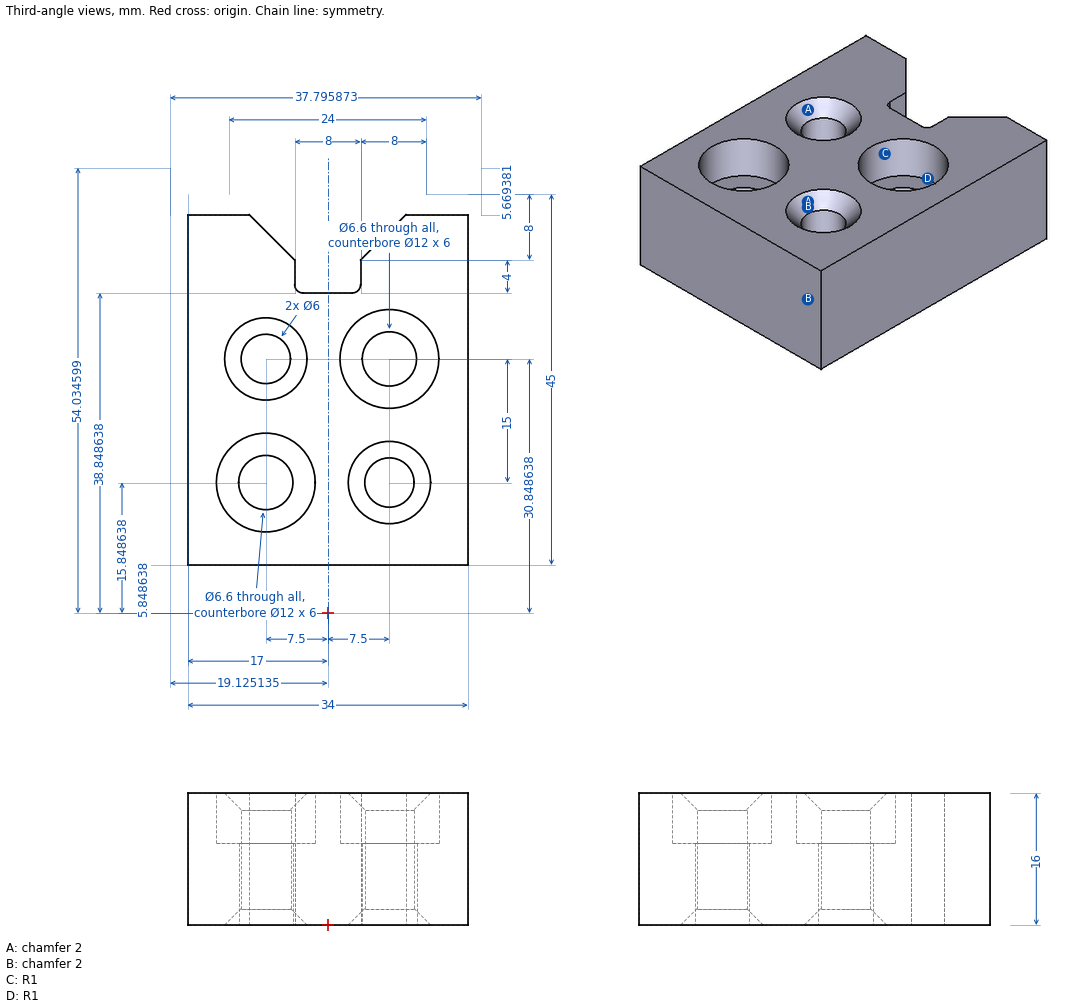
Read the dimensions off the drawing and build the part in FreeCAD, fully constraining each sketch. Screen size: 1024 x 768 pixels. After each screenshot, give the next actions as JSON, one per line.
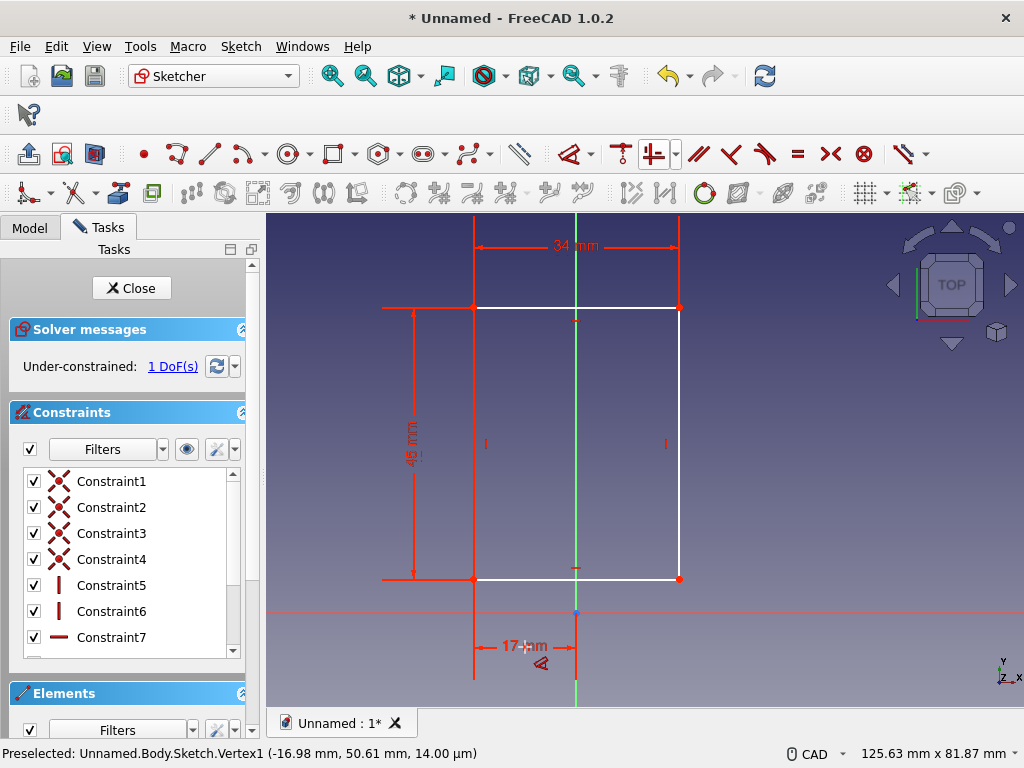
{"action": "left_click", "coordinate": [474, 580]}
{"action": "left_click", "coordinate": [440, 596]}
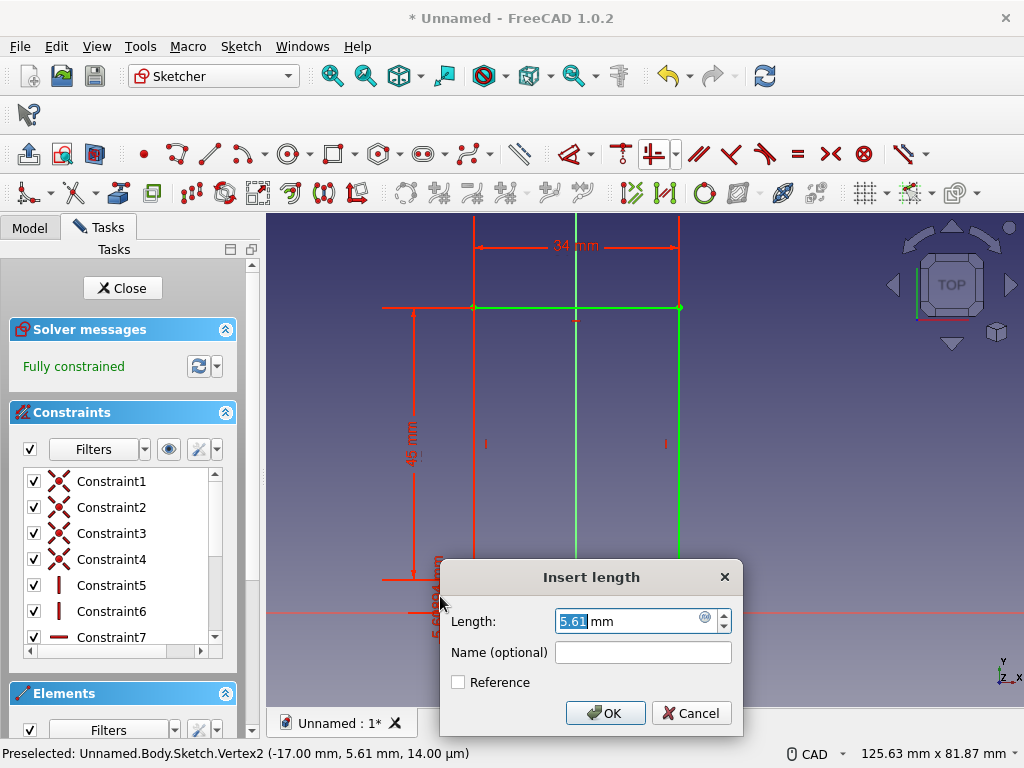
{"action": "type", "text": "5.848638"}
{"action": "key", "text": "Return"}
{"action": "key", "text": "Escape"}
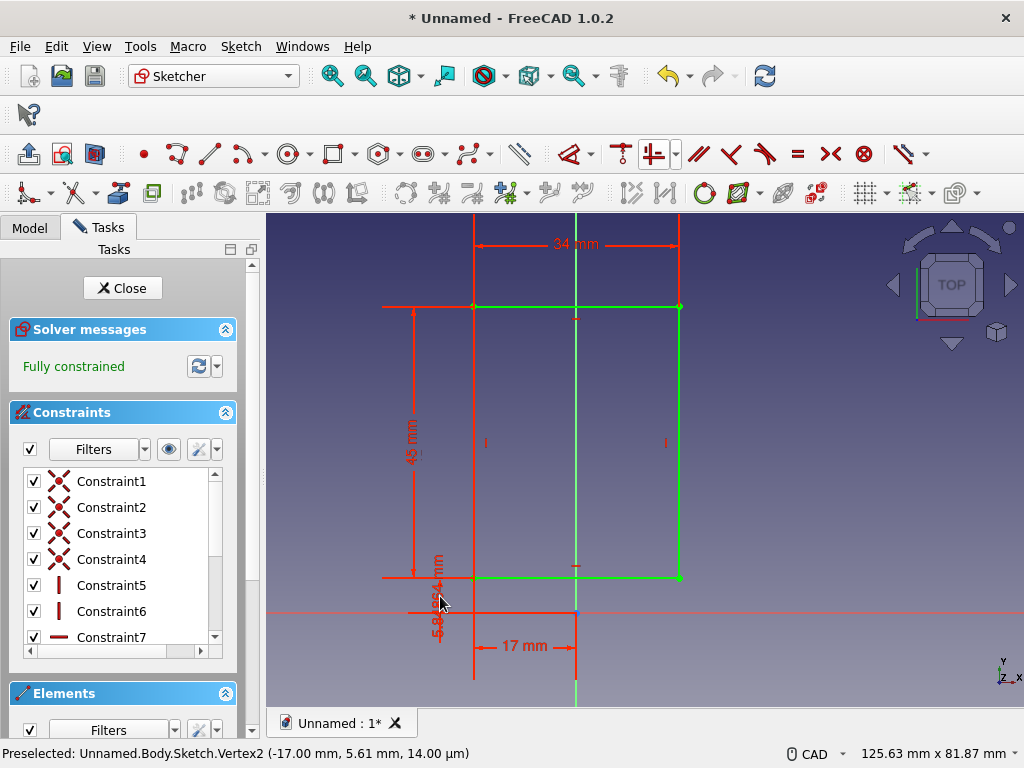
{"action": "left_click", "coordinate": [123, 288]}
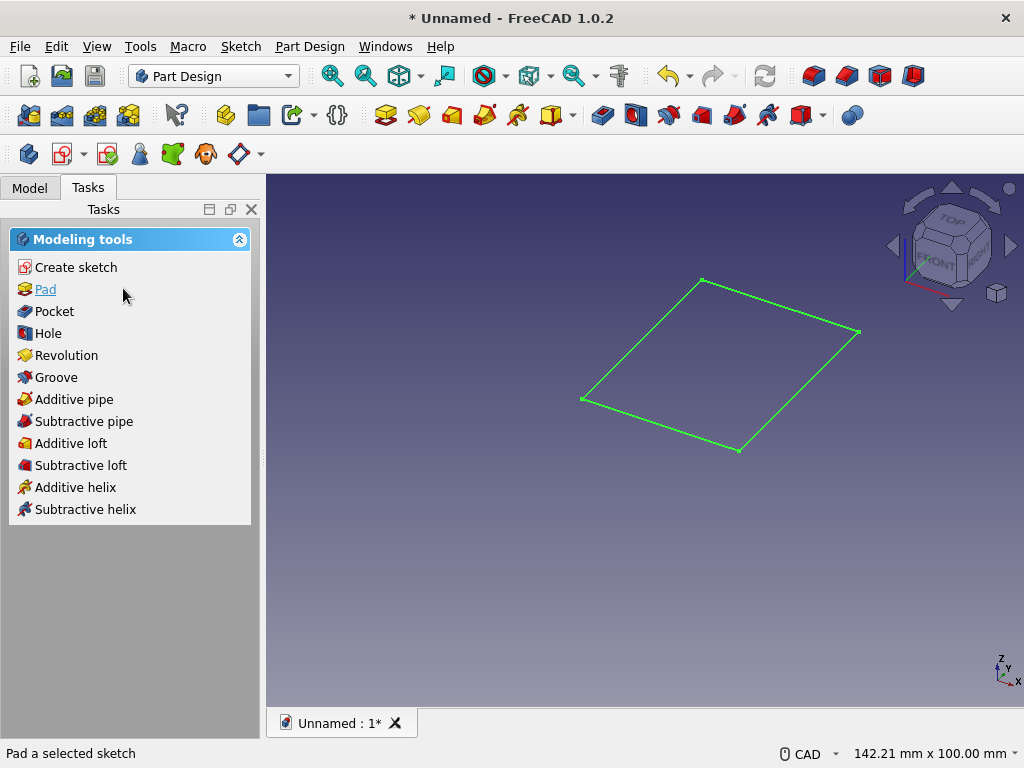
{"action": "left_click", "coordinate": [386, 116]}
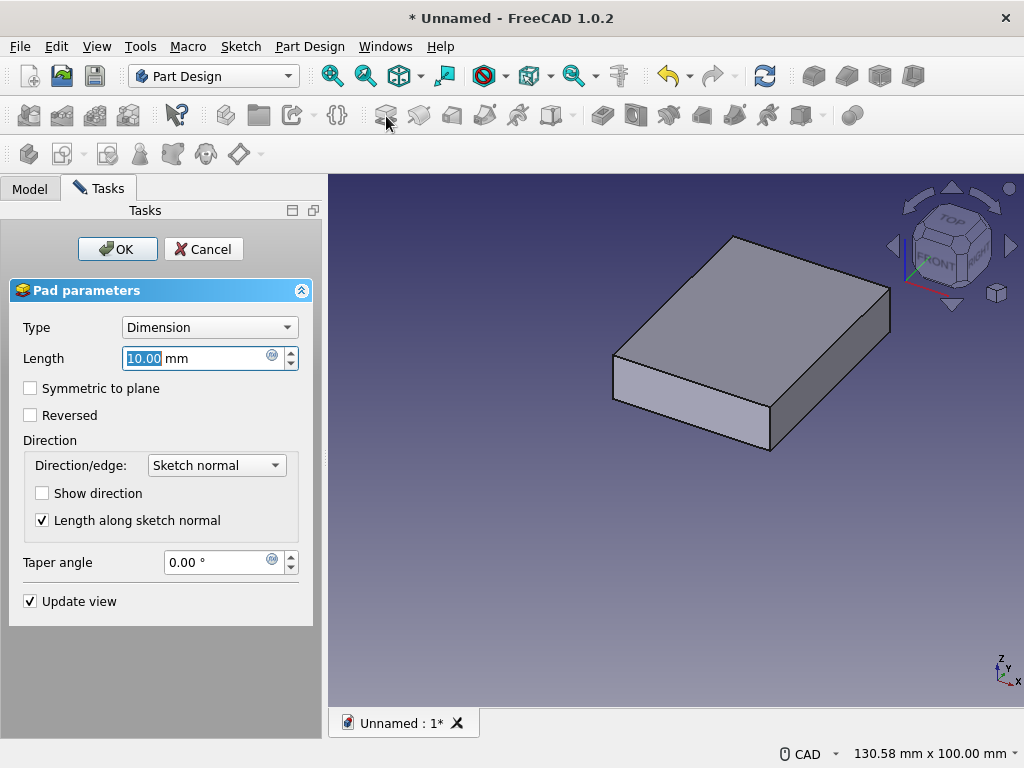
{"action": "type", "text": "16"}
{"action": "key", "text": "Tab"}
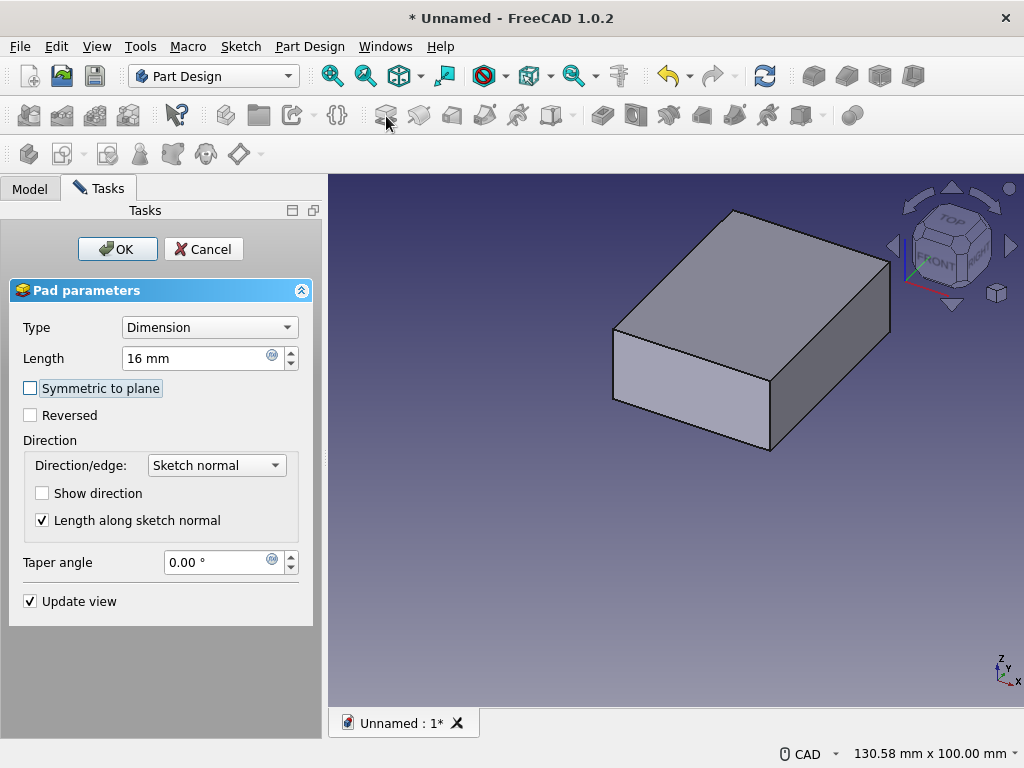
{"action": "left_click", "coordinate": [118, 249]}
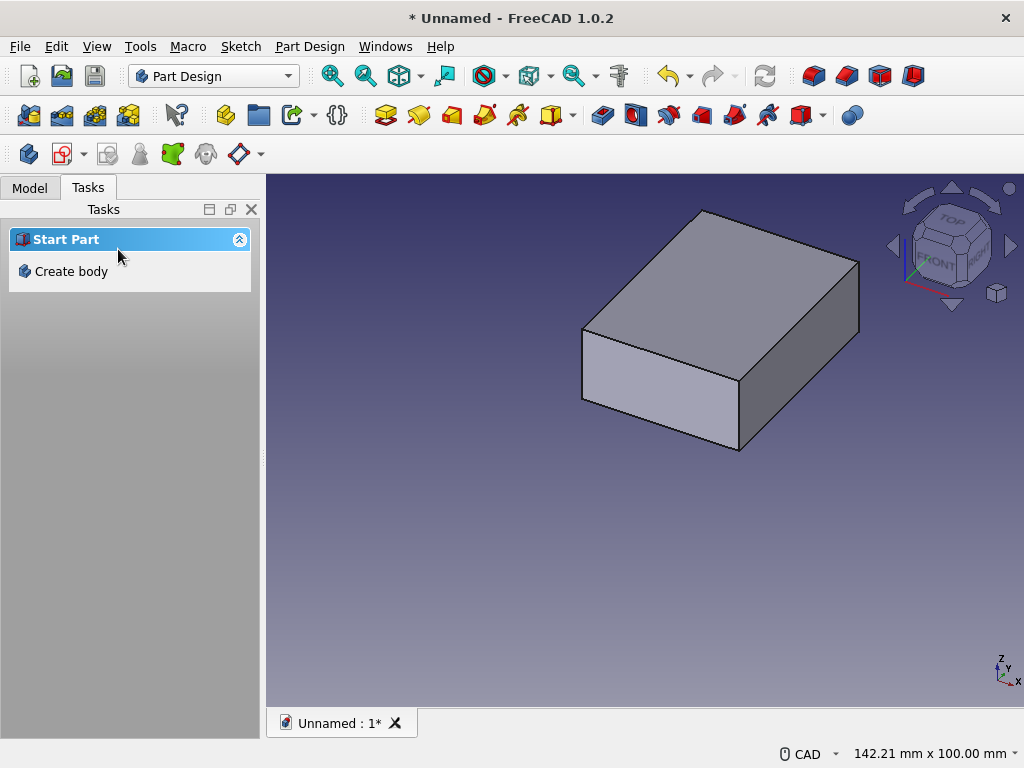
{"action": "left_click", "coordinate": [721, 295]}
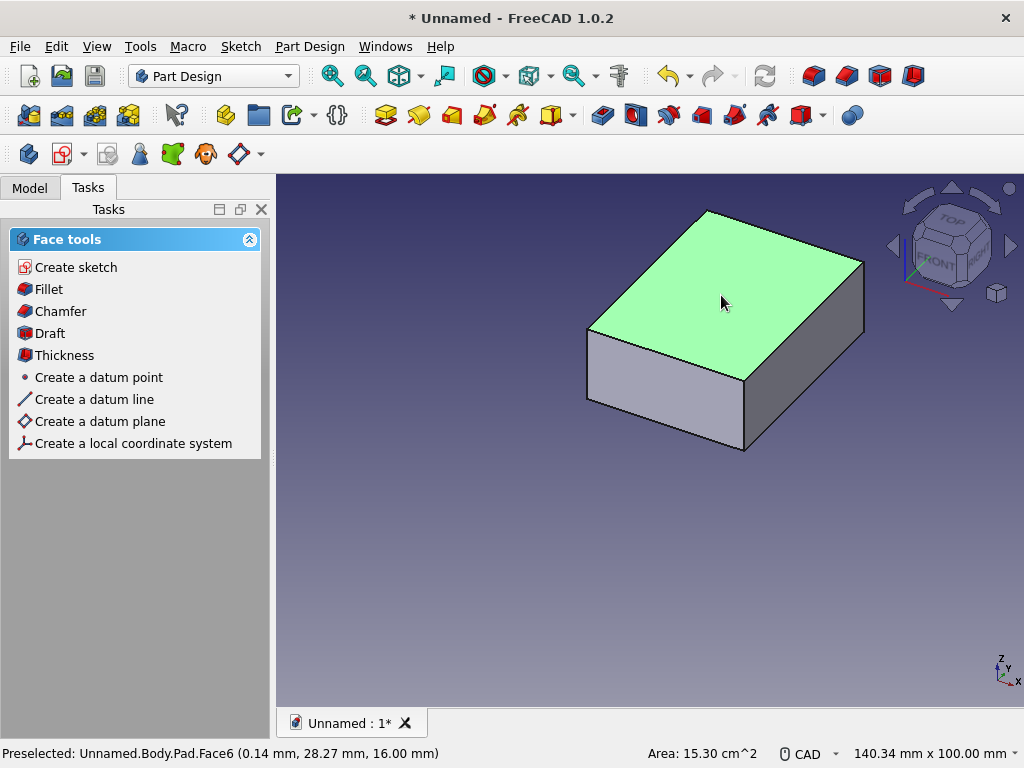
{"action": "left_click", "coordinate": [62, 154]}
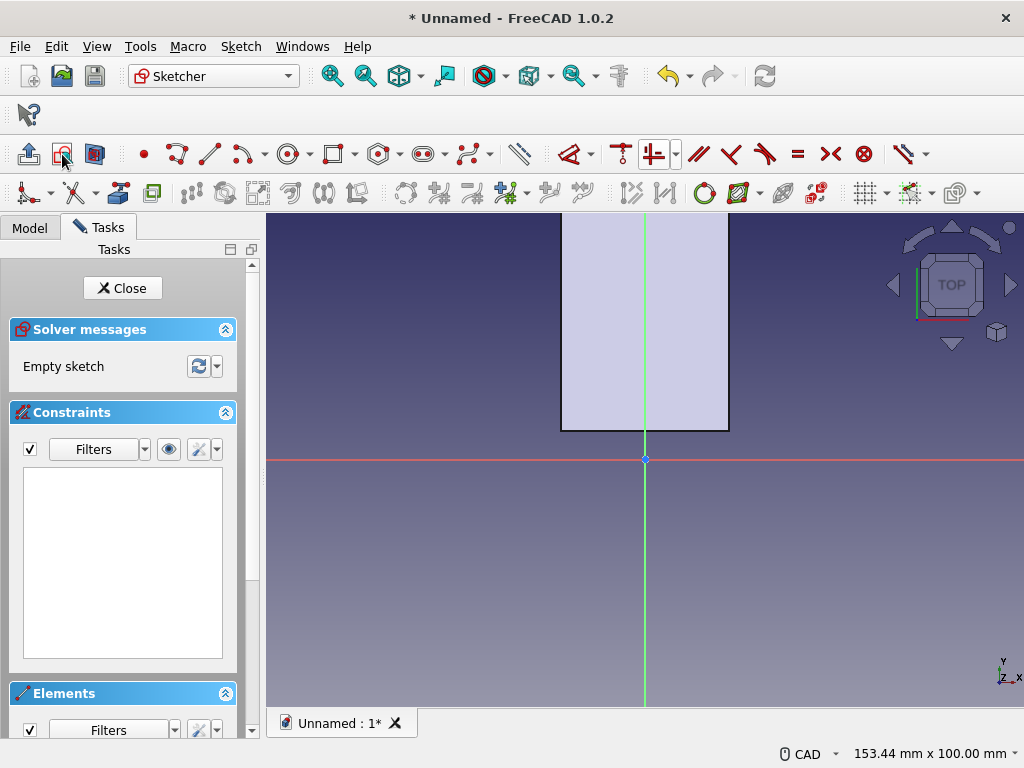
{"action": "scroll", "coordinate": [294, 679], "scroll_direction": "down", "scroll_amount": 1}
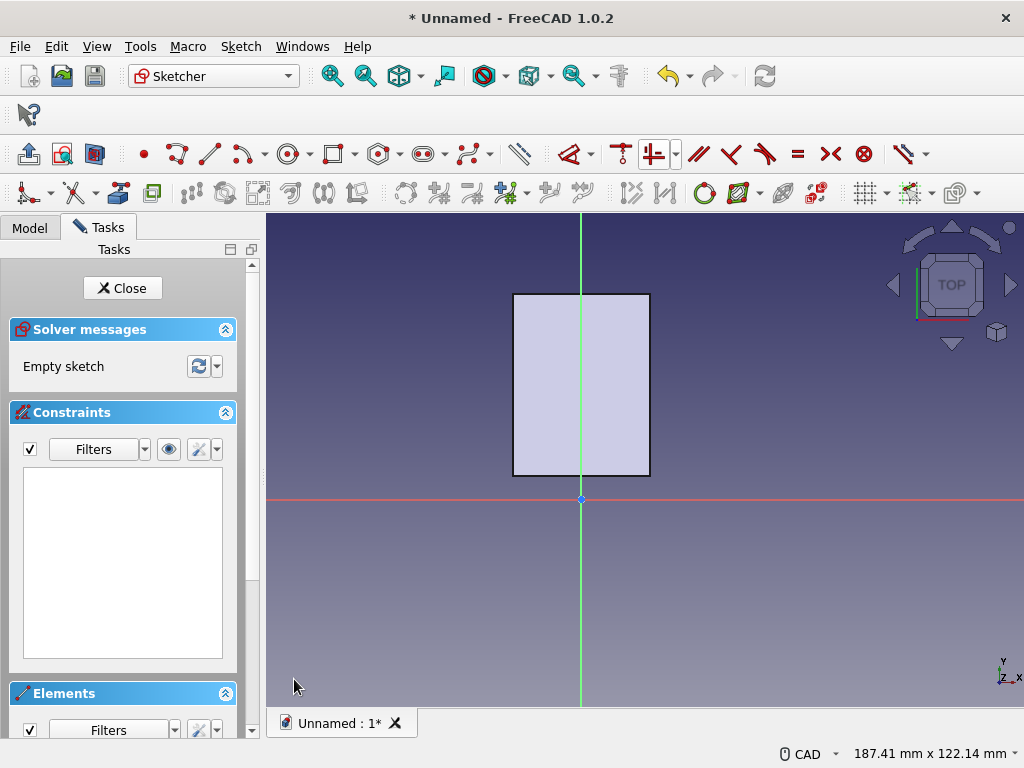
{"action": "scroll", "coordinate": [591, 269], "scroll_direction": "up", "scroll_amount": 2}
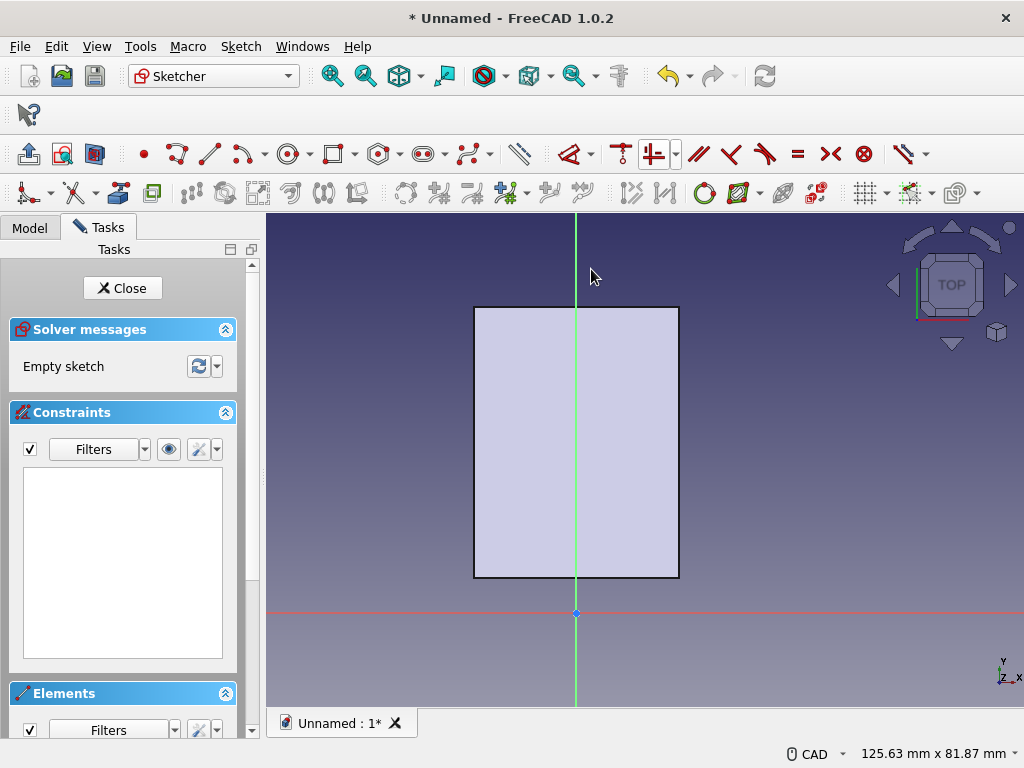
{"action": "left_click", "coordinate": [177, 154]}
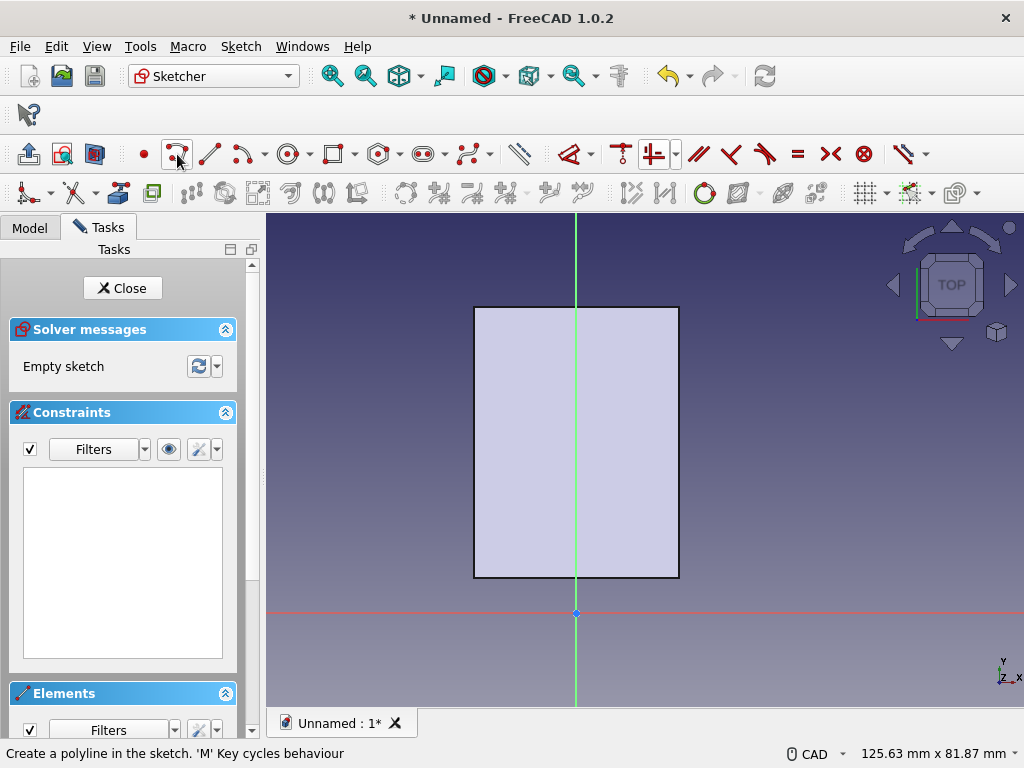
{"action": "left_click", "coordinate": [552, 379]}
{"action": "left_click", "coordinate": [601, 379]}
{"action": "left_click", "coordinate": [601, 355]}
{"action": "left_click", "coordinate": [649, 307]}
{"action": "left_click", "coordinate": [504, 307]}
{"action": "left_click", "coordinate": [552, 355]}
{"action": "left_click", "coordinate": [552, 380]}
{"action": "key", "text": "Escape"}
{"action": "key", "text": "Escape"}